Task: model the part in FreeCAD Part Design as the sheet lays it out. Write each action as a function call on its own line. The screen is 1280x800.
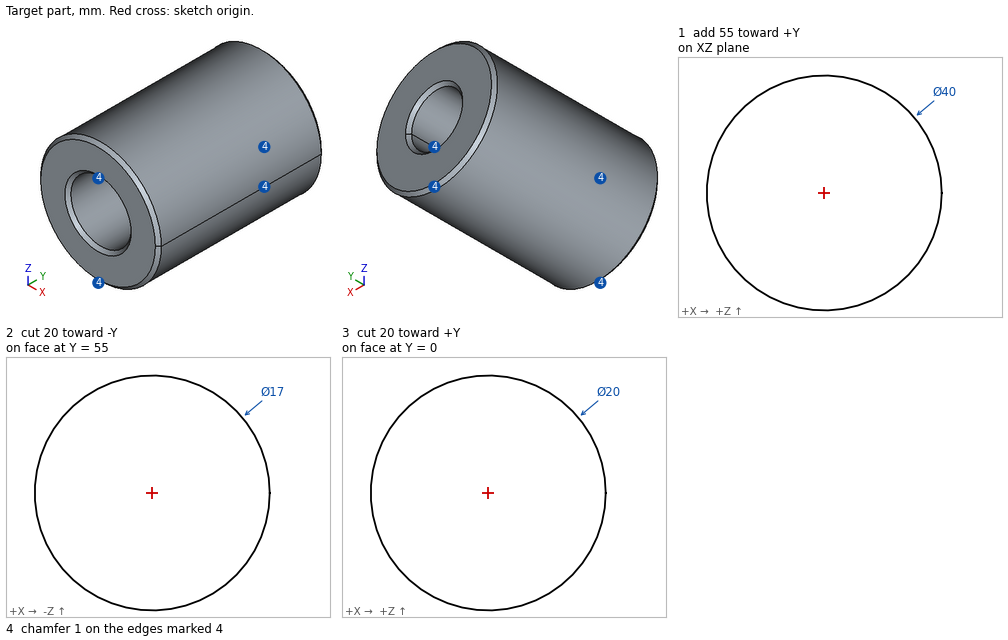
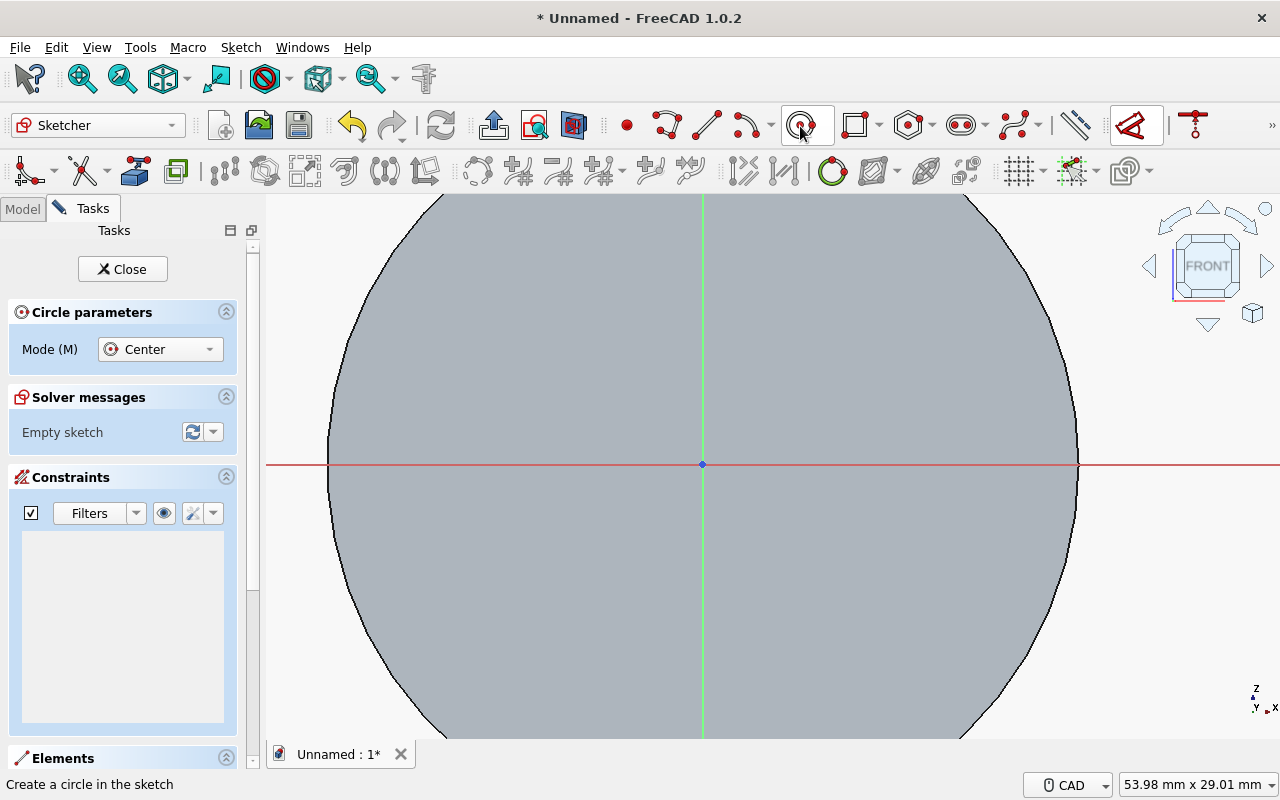
click(703, 465)
move(836, 332)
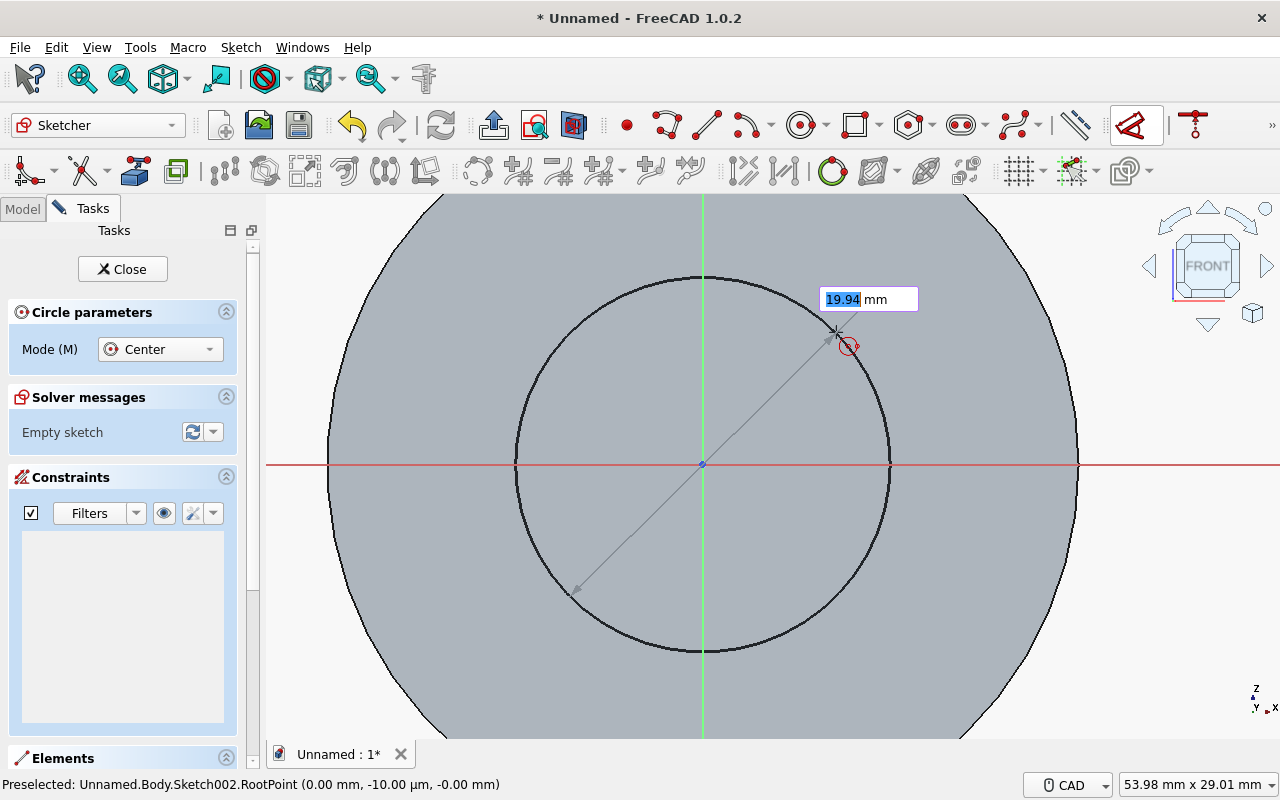
text(20)
key(Return)
key(Escape)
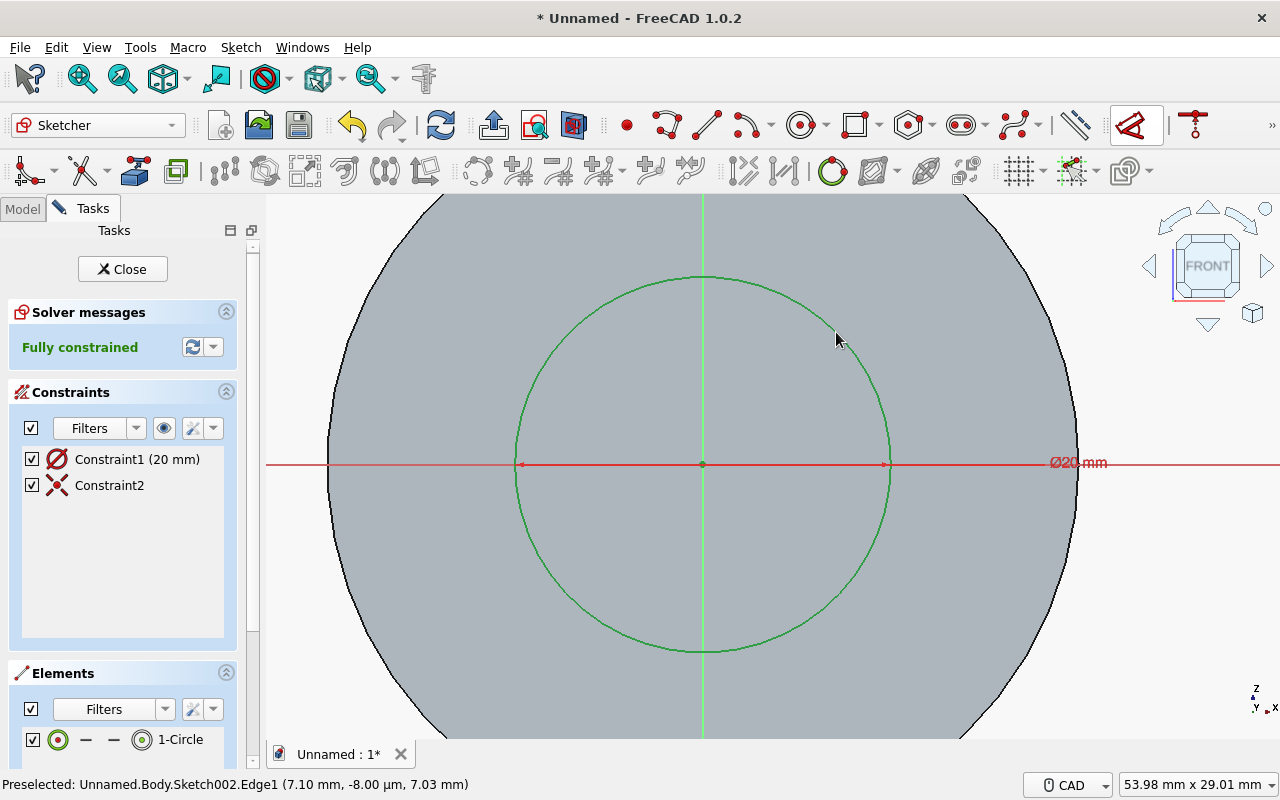
click(123, 269)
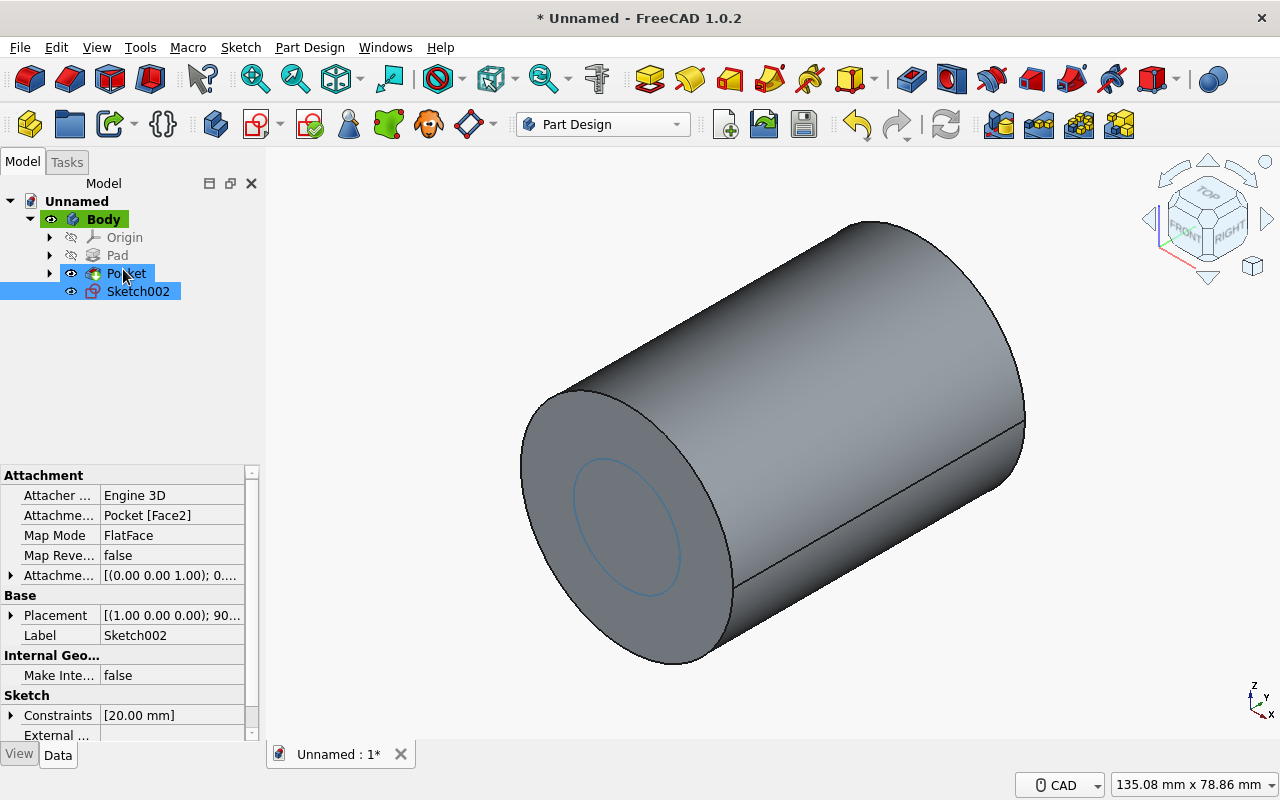
click(912, 80)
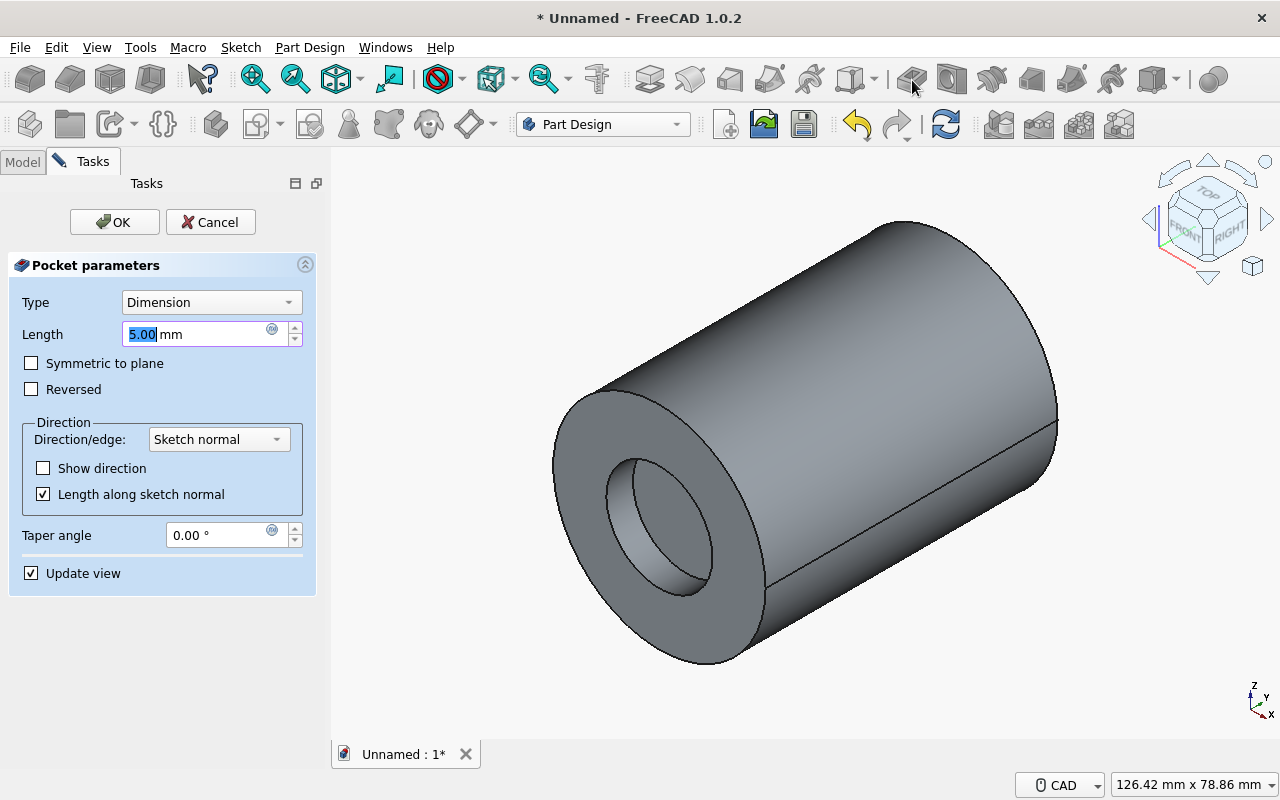
text(20)
key(Tab)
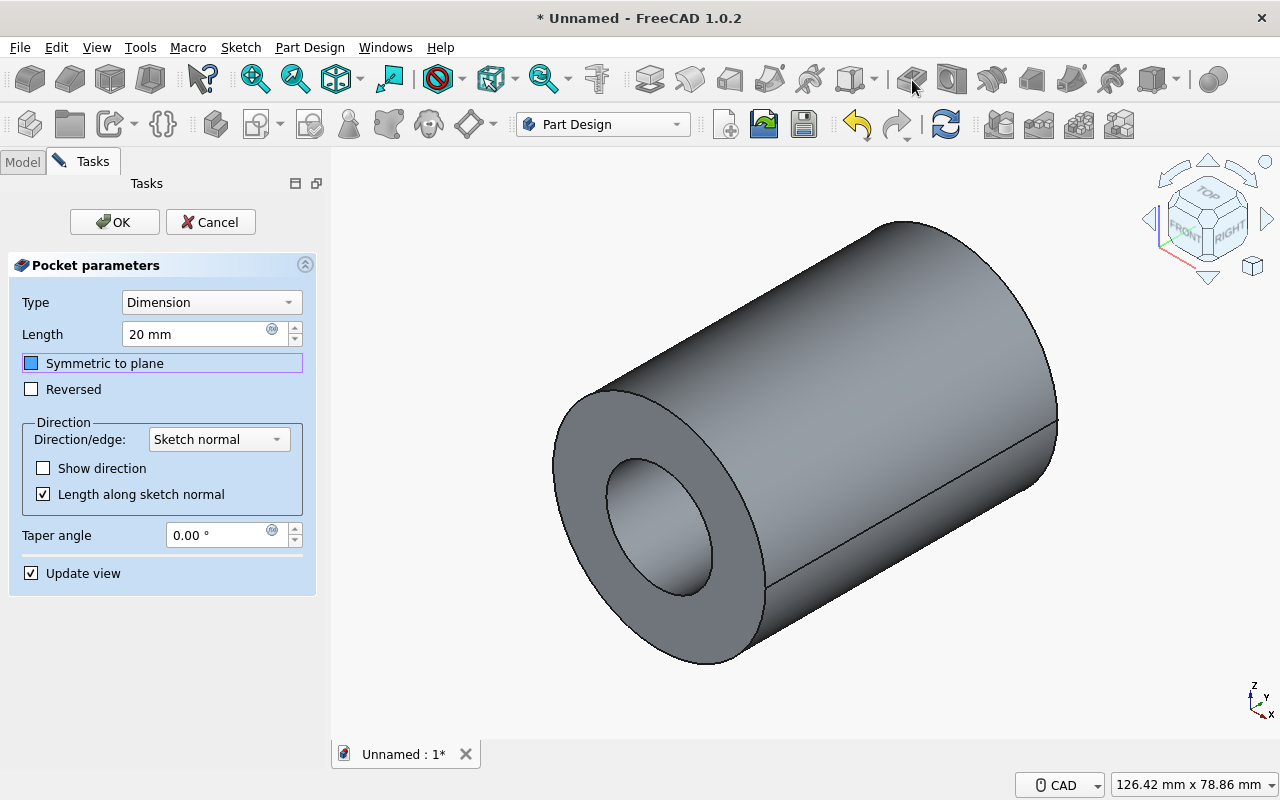
click(115, 222)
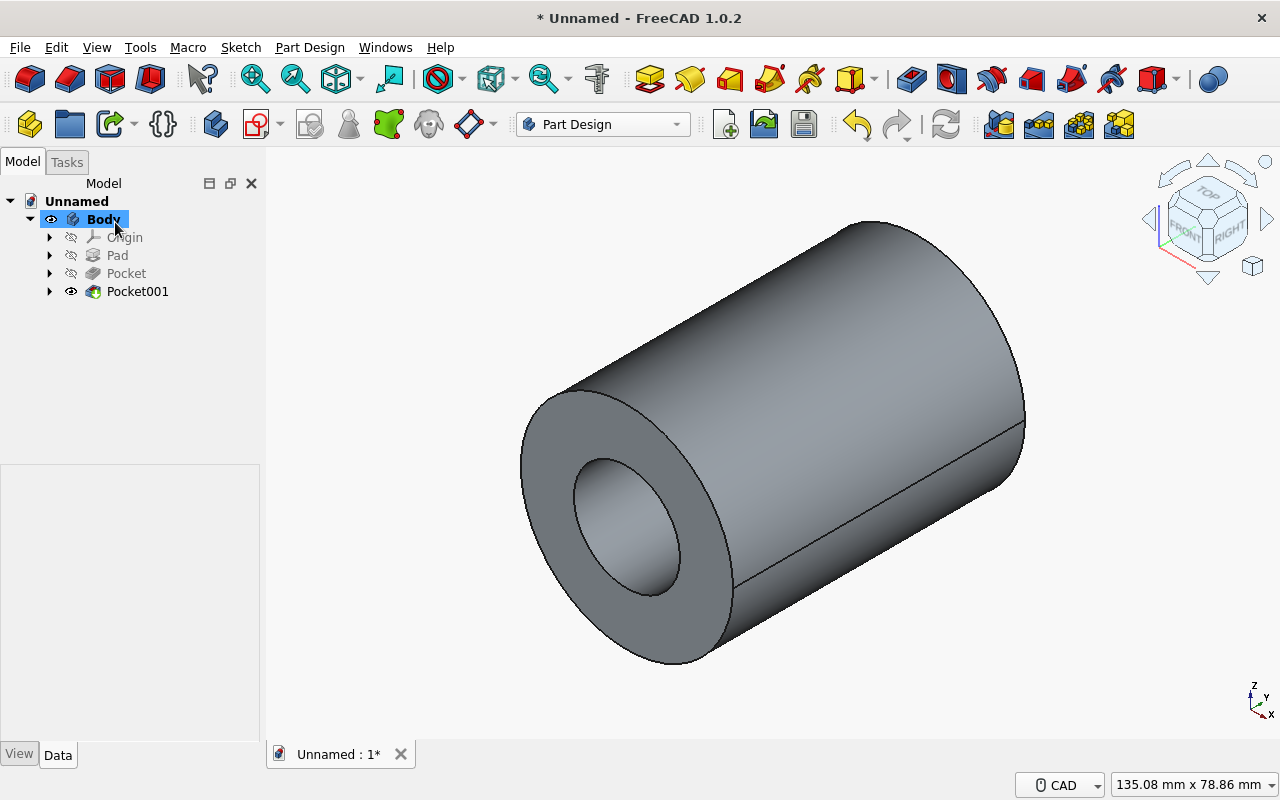
click(574, 496)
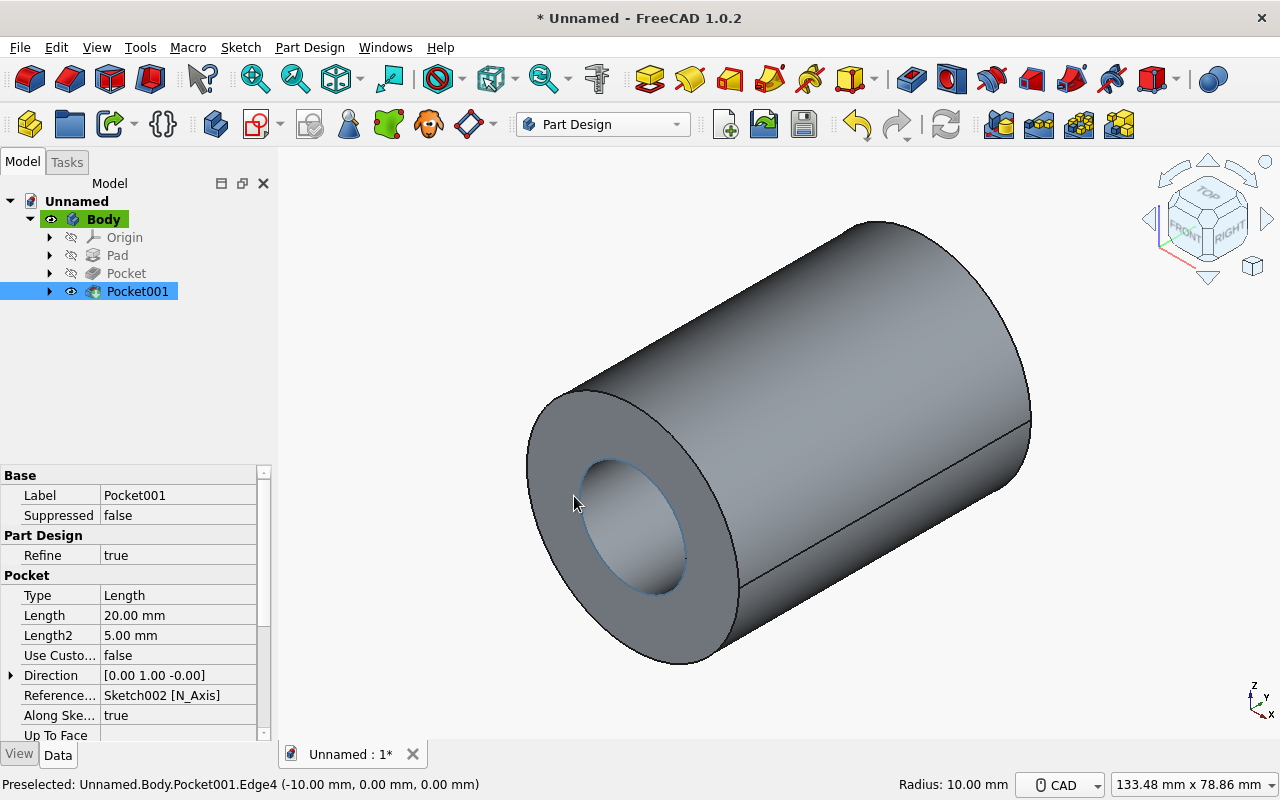
click(600, 391, ctrl)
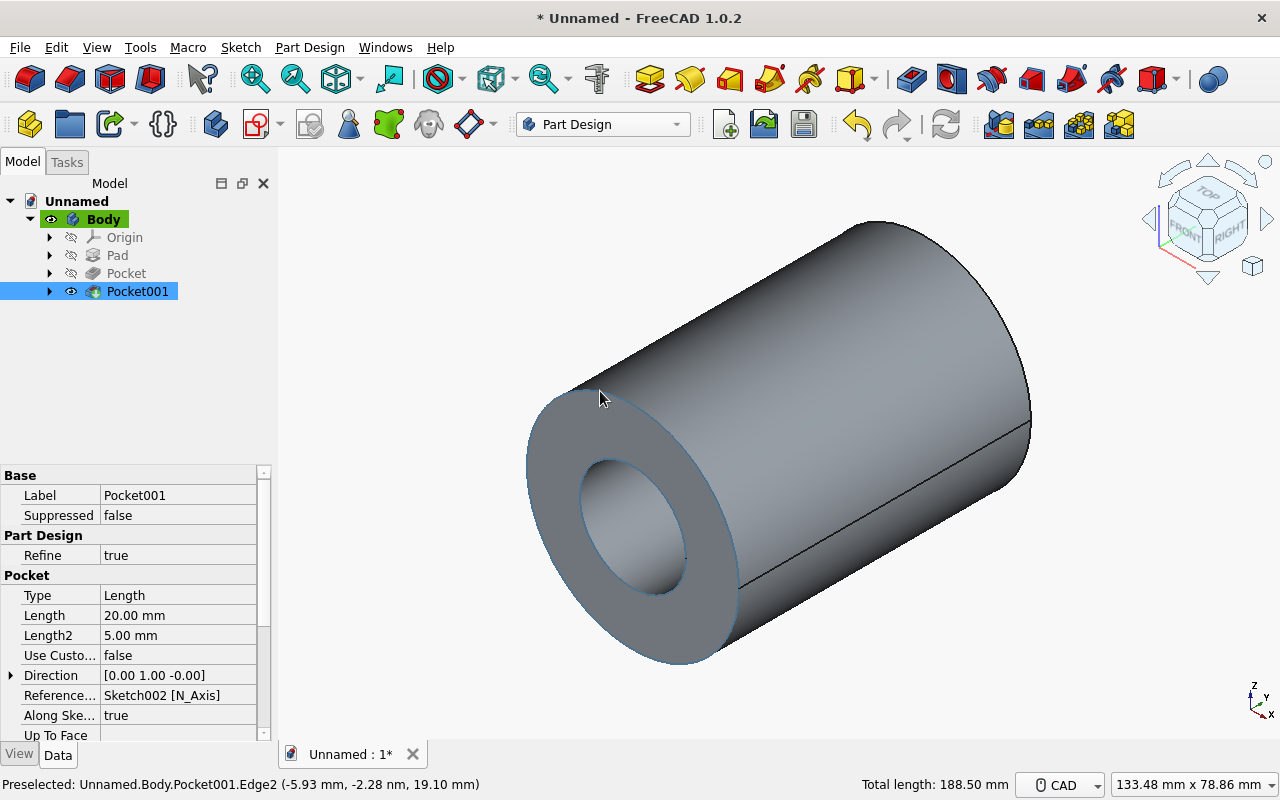
key(2)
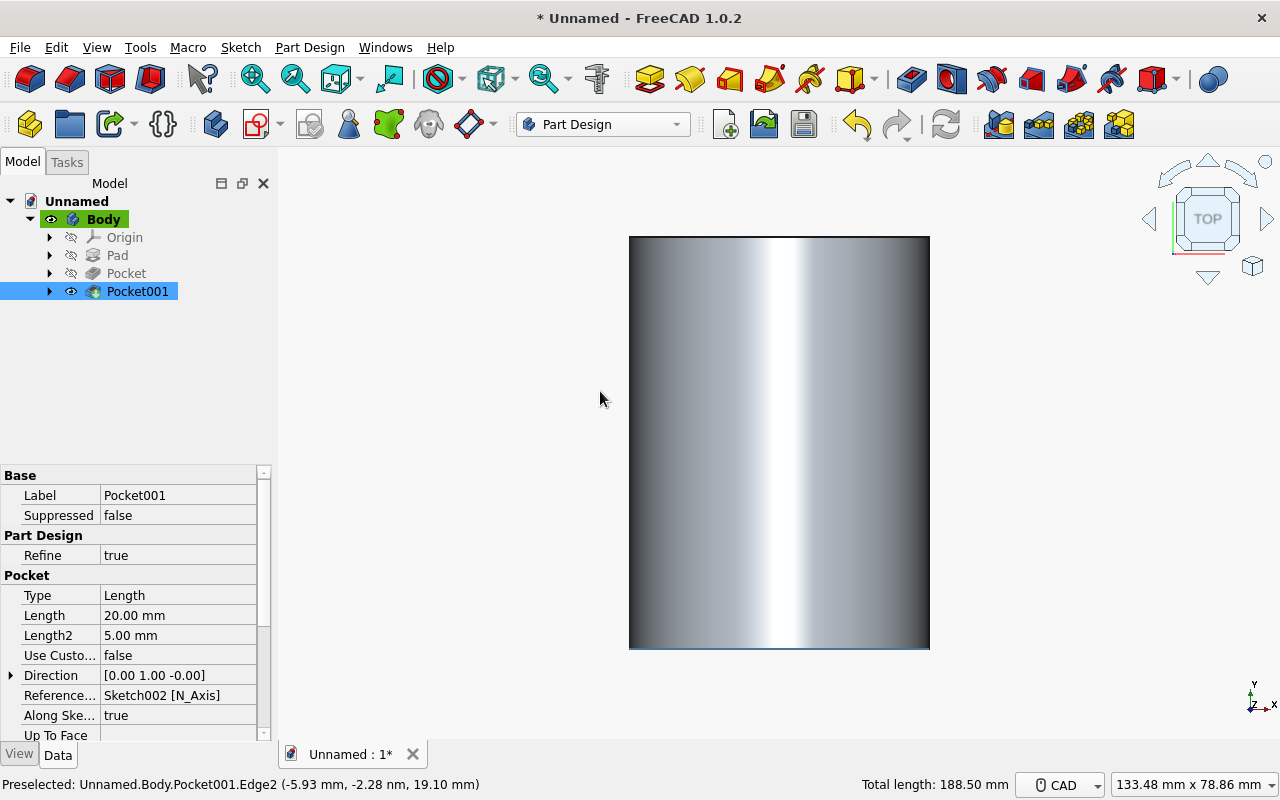
click(657, 236, ctrl)